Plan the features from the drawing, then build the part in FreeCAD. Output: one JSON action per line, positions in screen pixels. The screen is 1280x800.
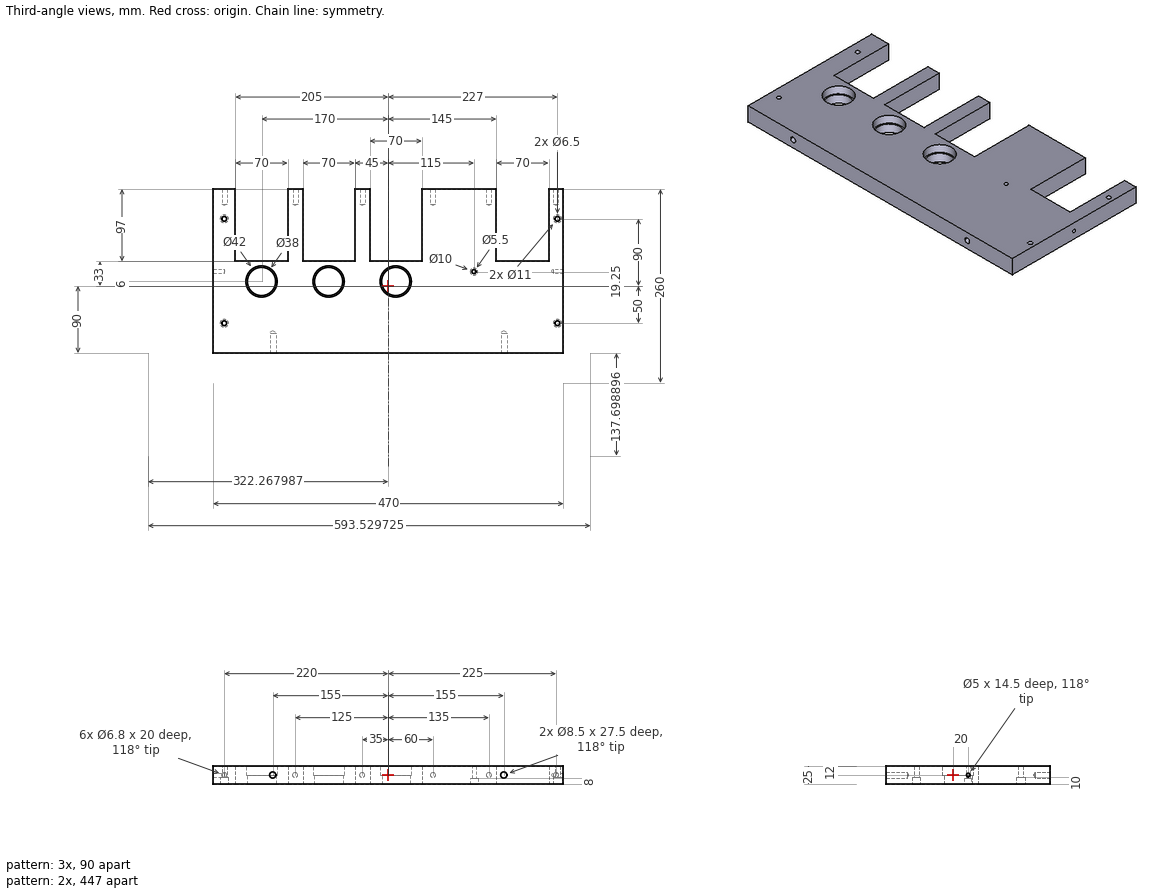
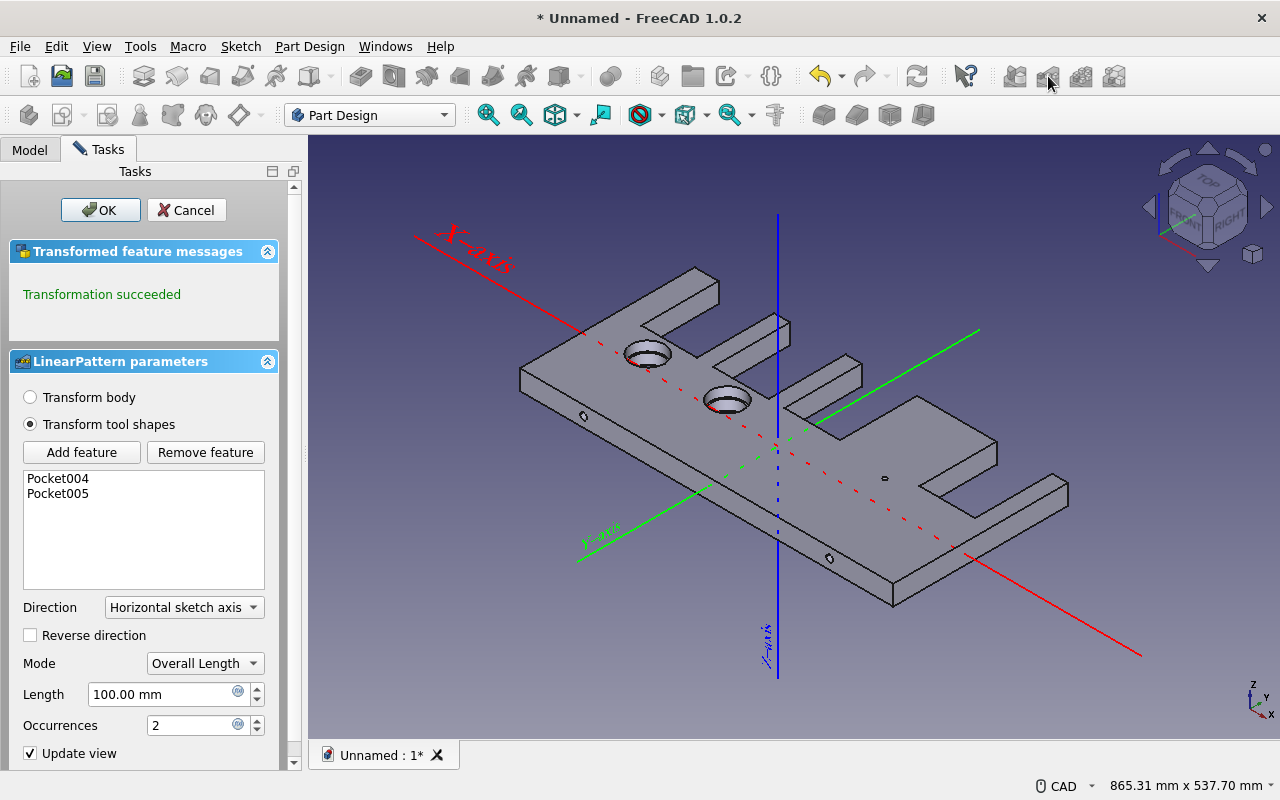
{"action": "left_click", "coordinate": [185, 608]}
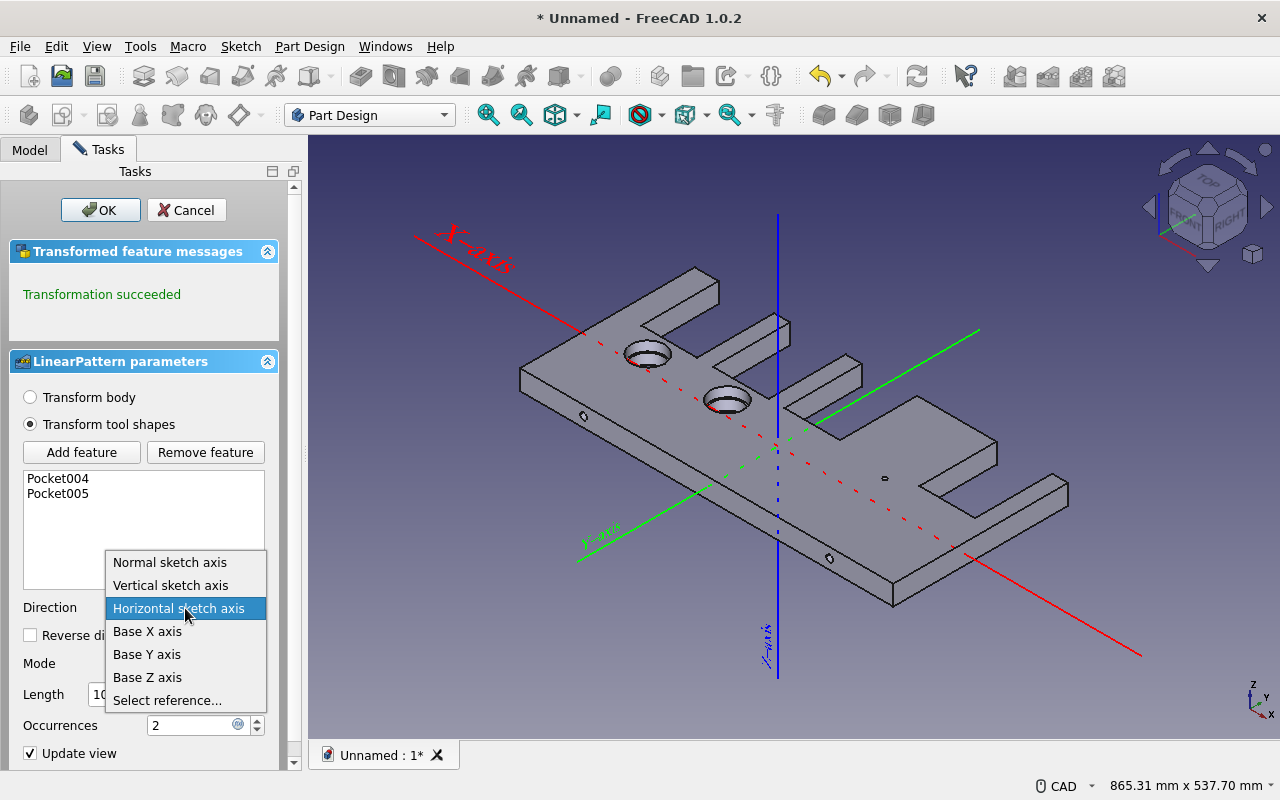
{"action": "left_click", "coordinate": [184, 632]}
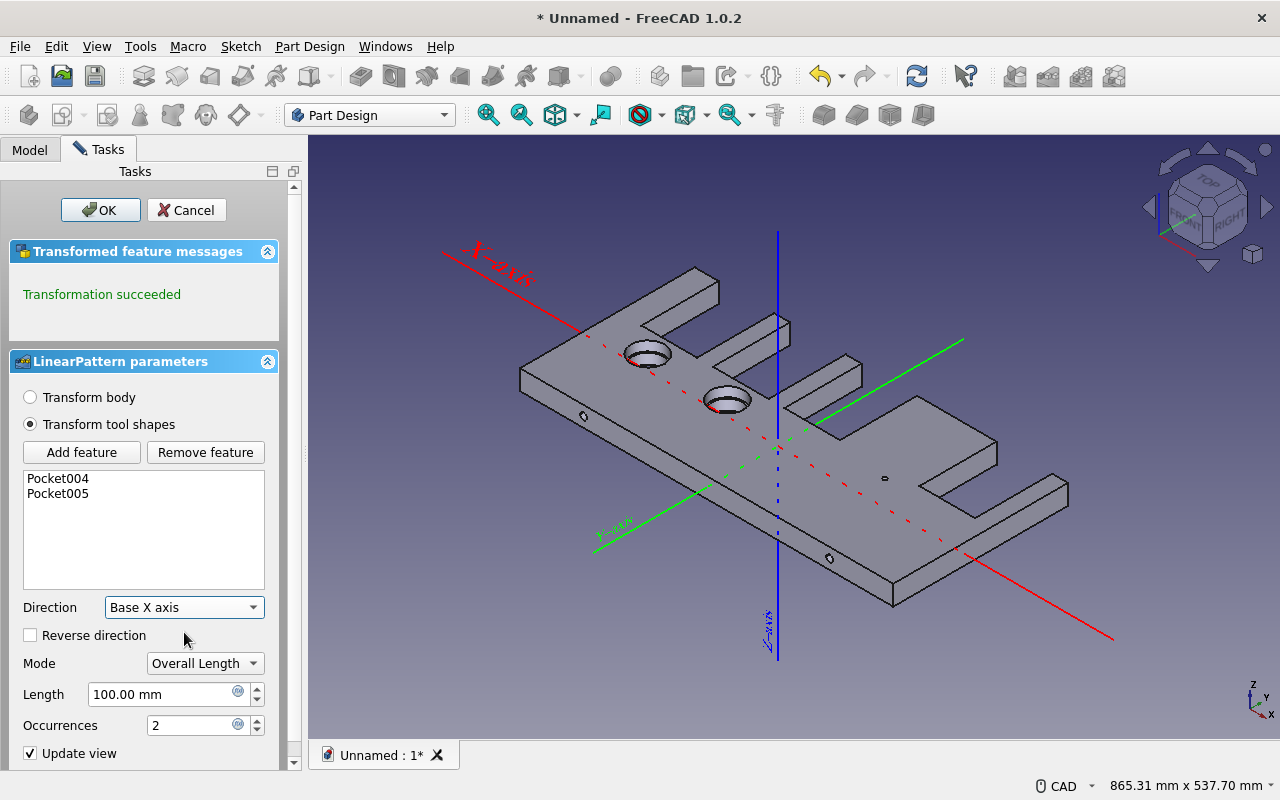
{"action": "left_click", "coordinate": [206, 664]}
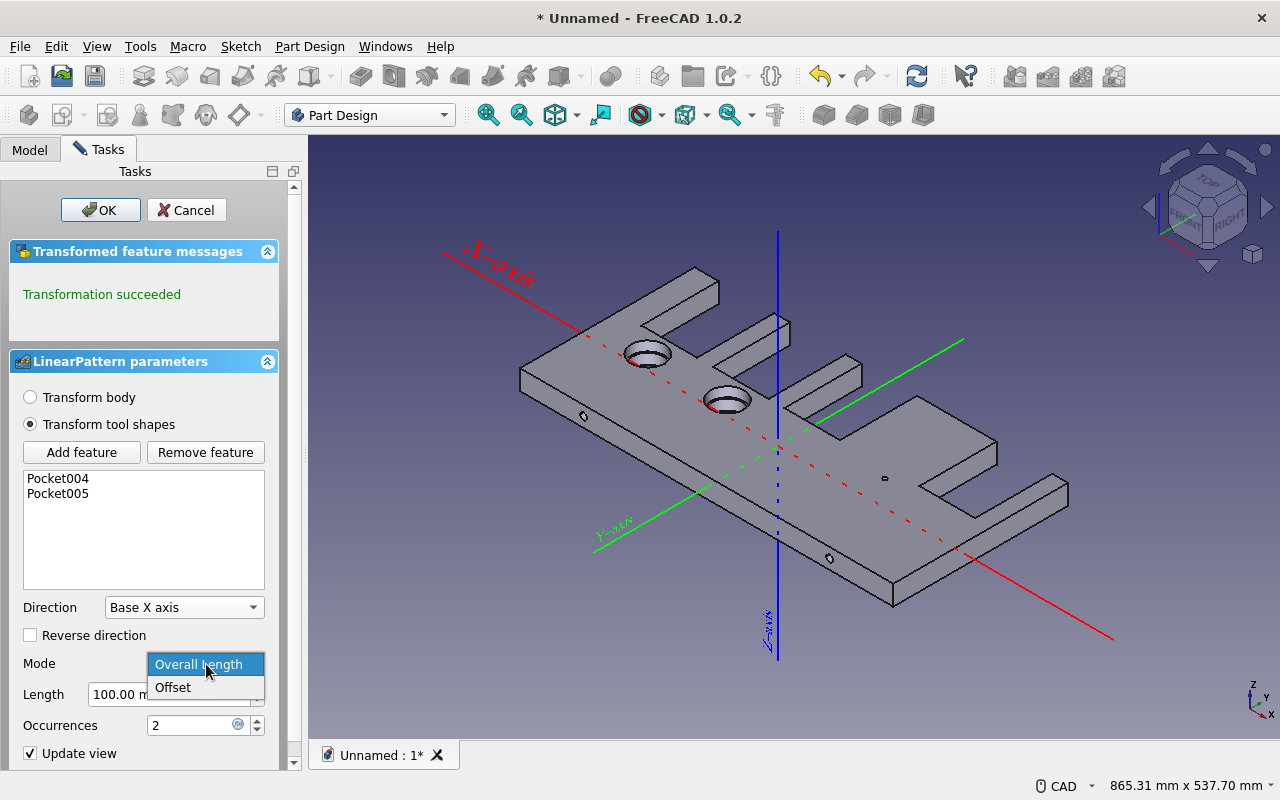
{"action": "left_click", "coordinate": [204, 688]}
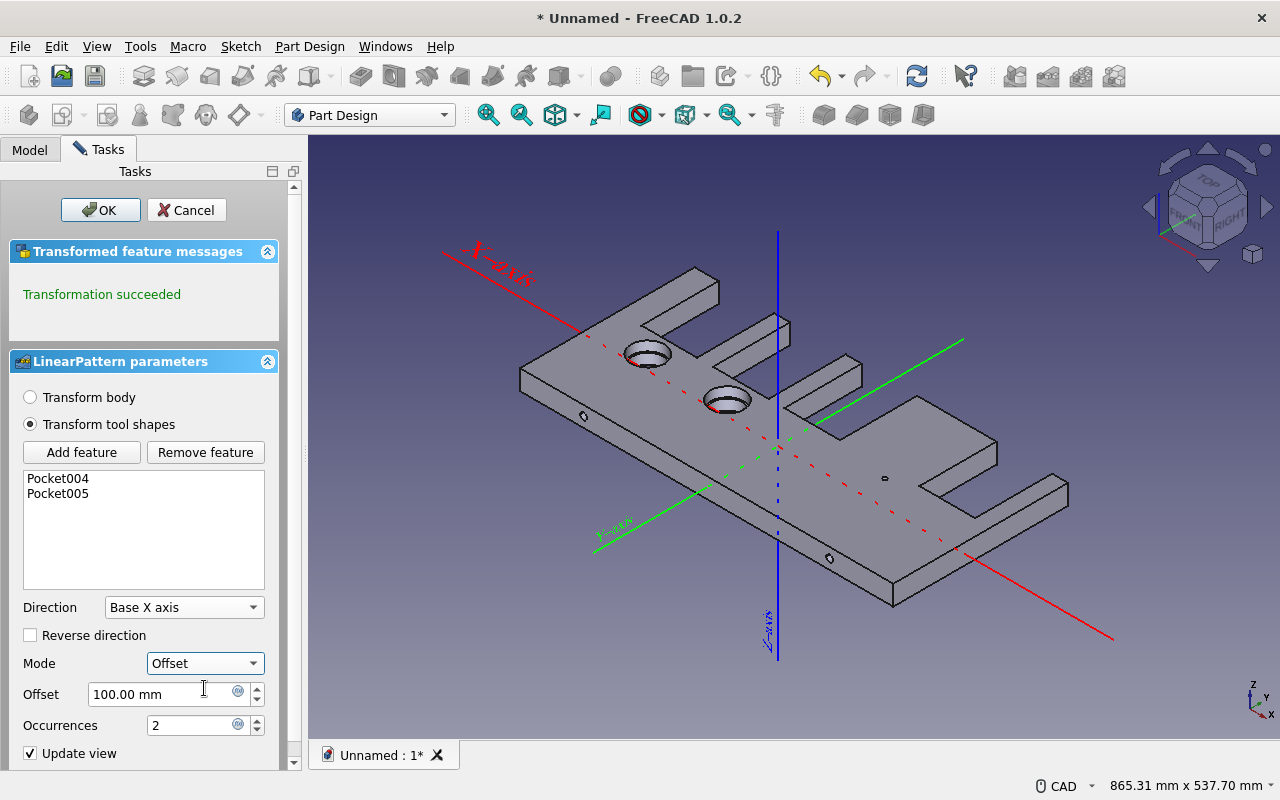
{"action": "triple_click", "coordinate": [170, 694]}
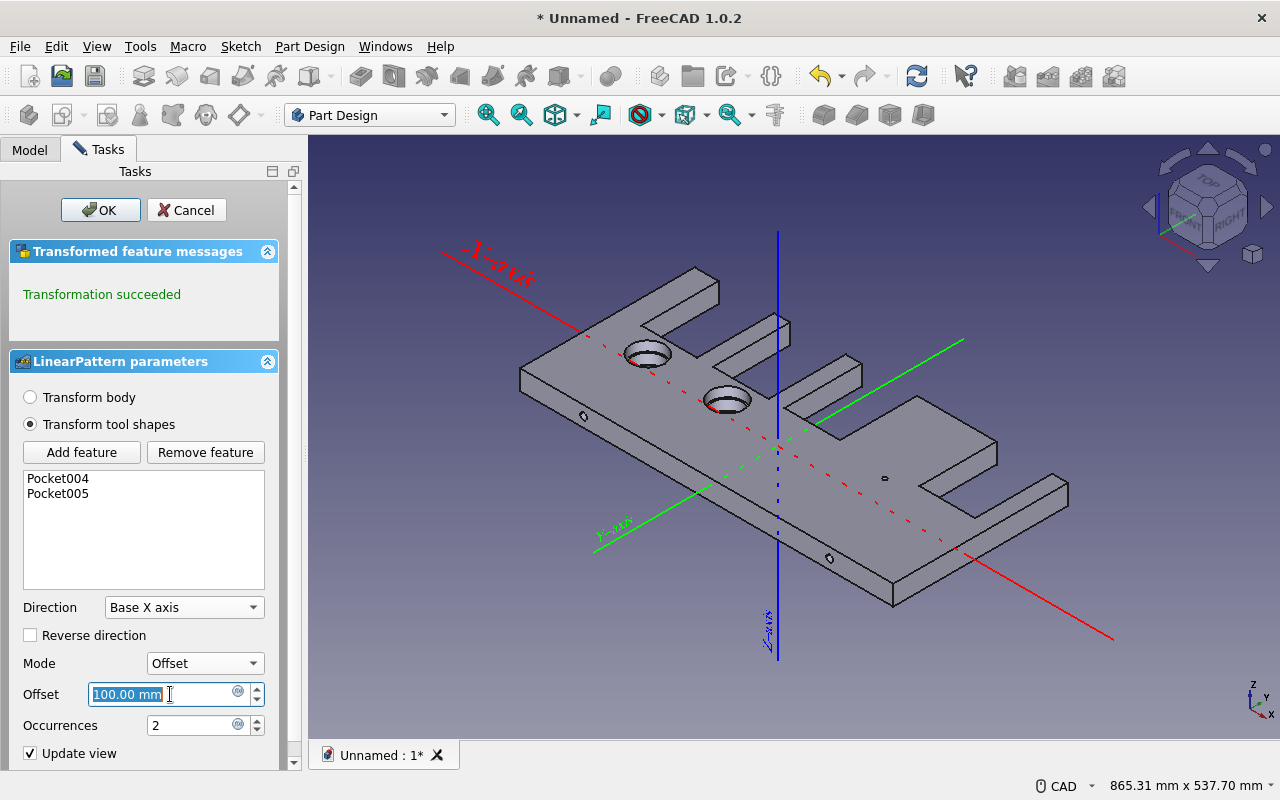
{"action": "type", "text": "90"}
{"action": "key", "text": "Tab"}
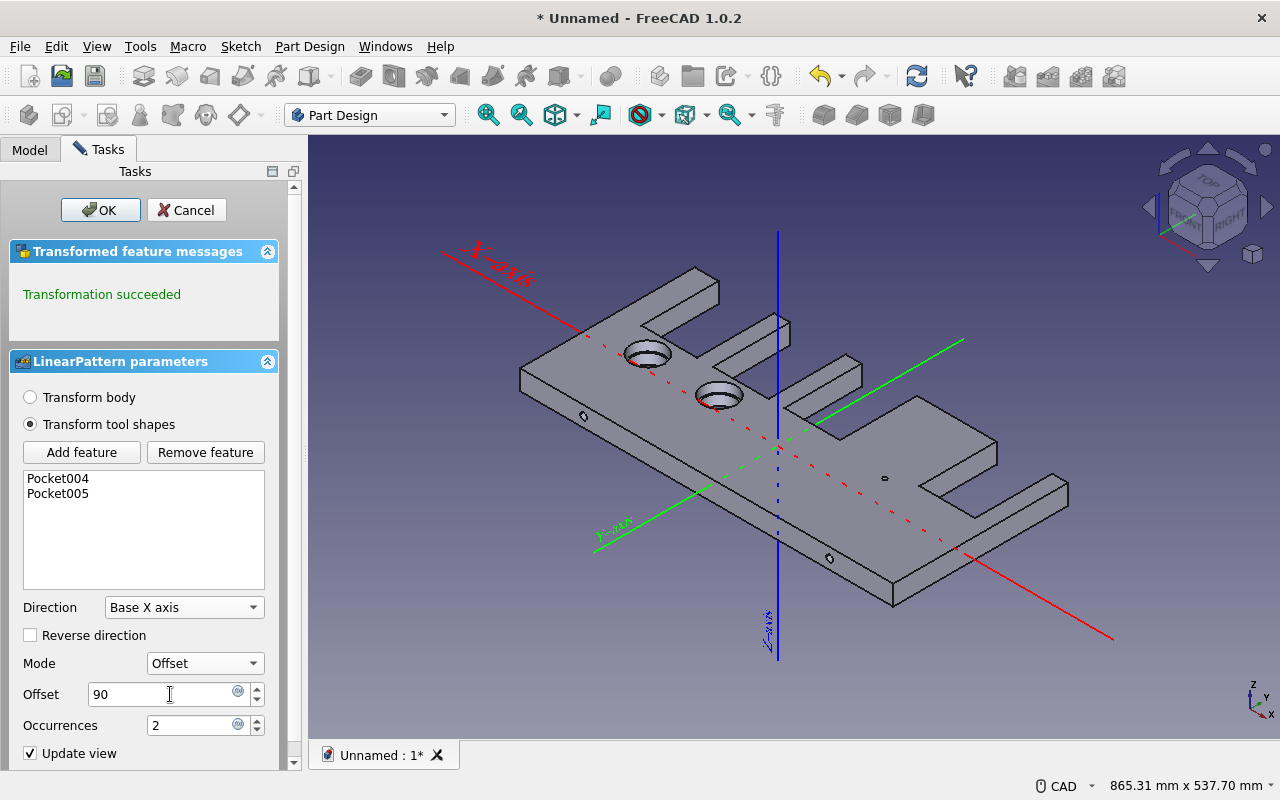
{"action": "triple_click", "coordinate": [199, 726]}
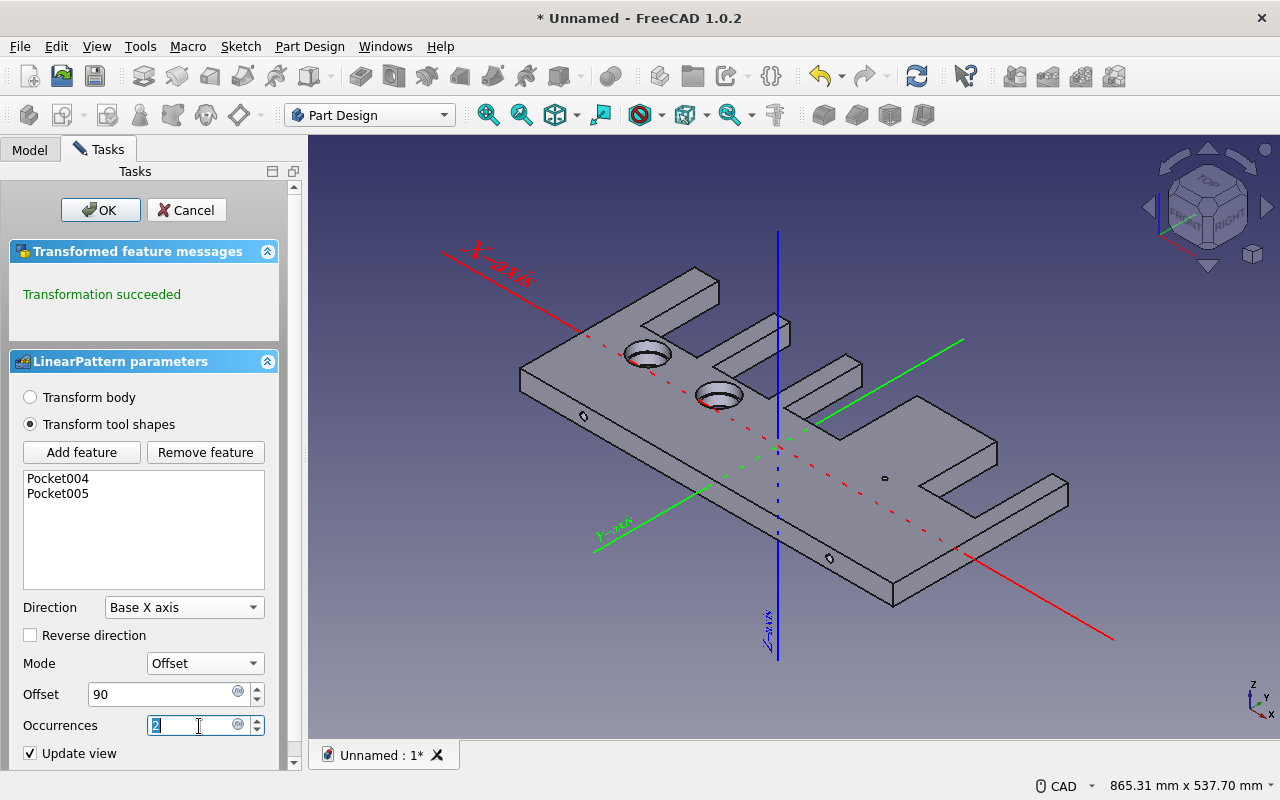
{"action": "type", "text": "3"}
{"action": "key", "text": "Tab"}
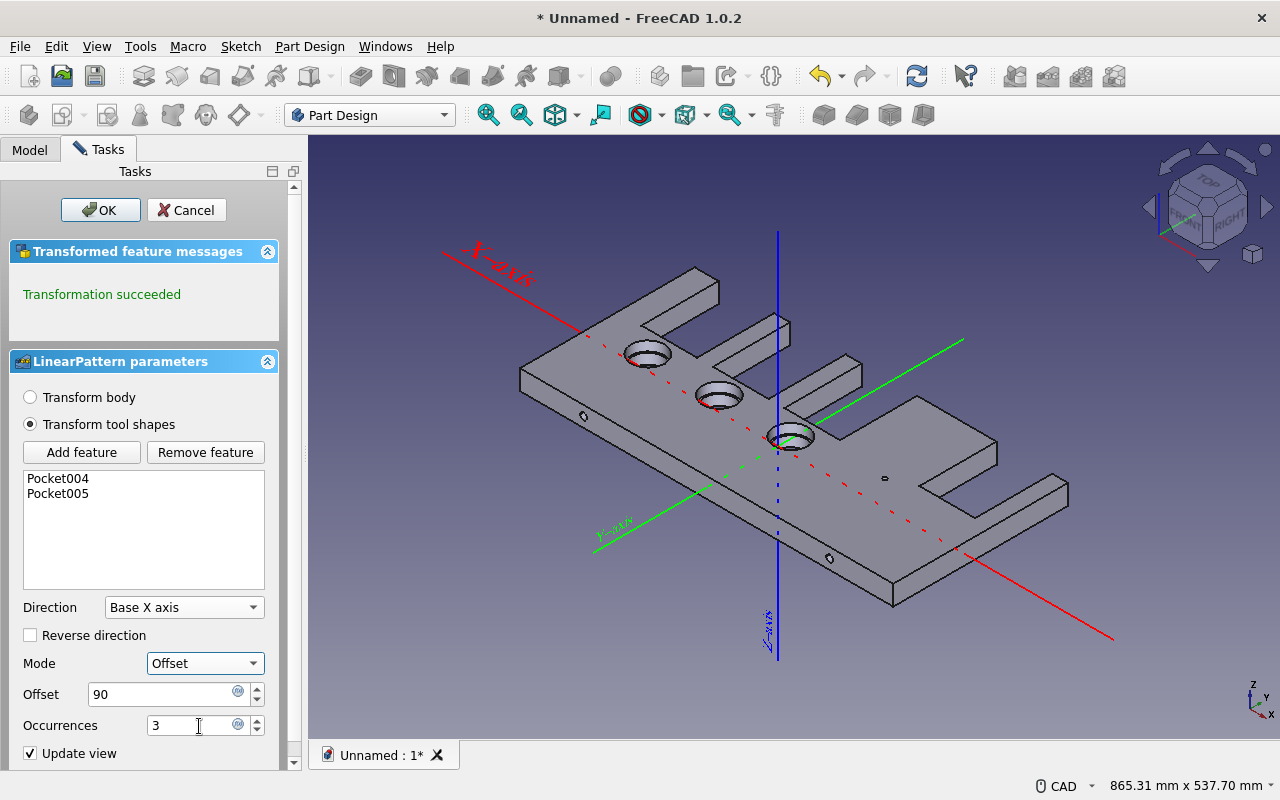
{"action": "left_click", "coordinate": [101, 210]}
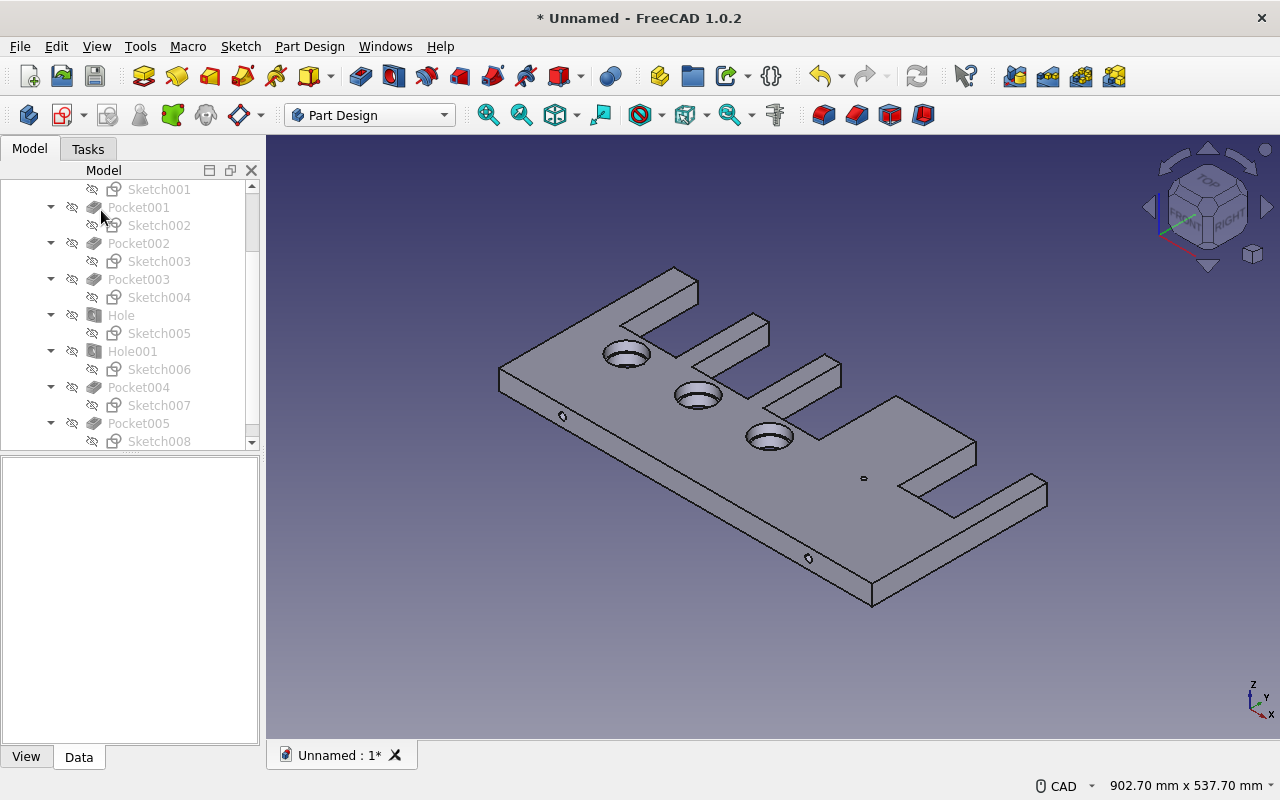
{"action": "key", "text": "5"}